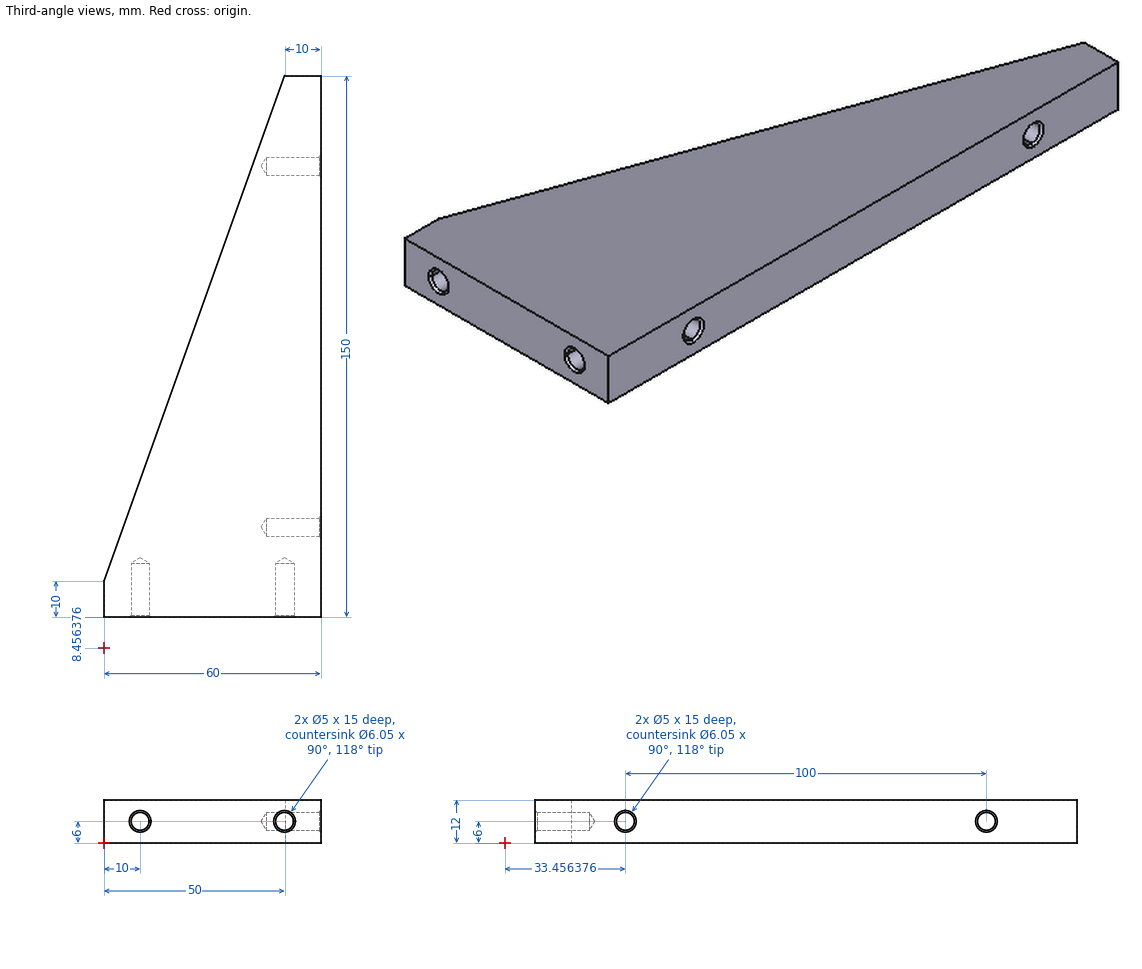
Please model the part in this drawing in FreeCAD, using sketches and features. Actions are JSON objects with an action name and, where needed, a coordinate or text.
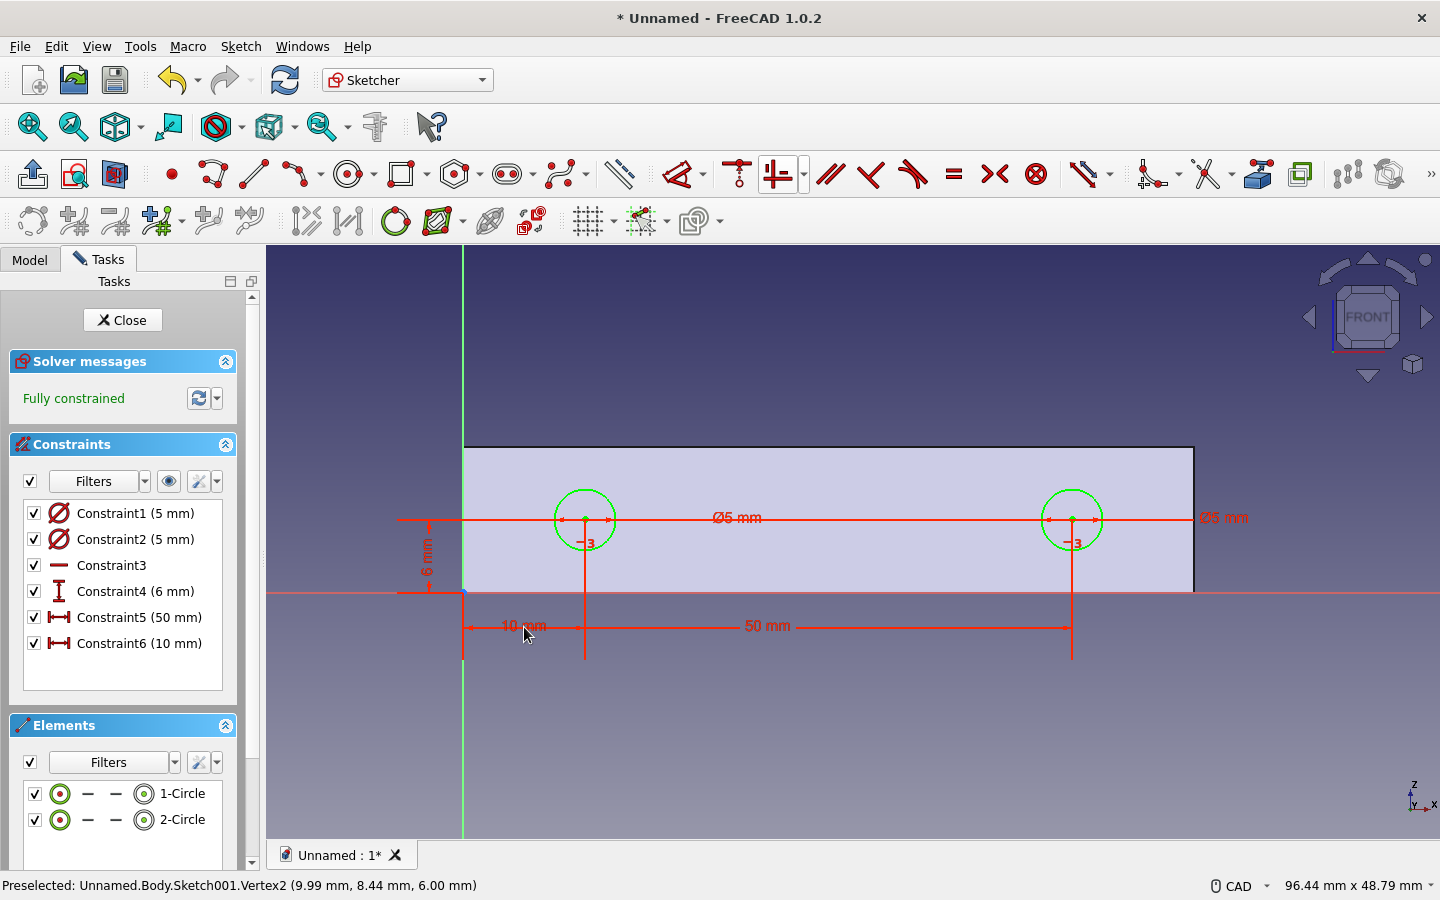
{"action": "left_click", "coordinate": [123, 320]}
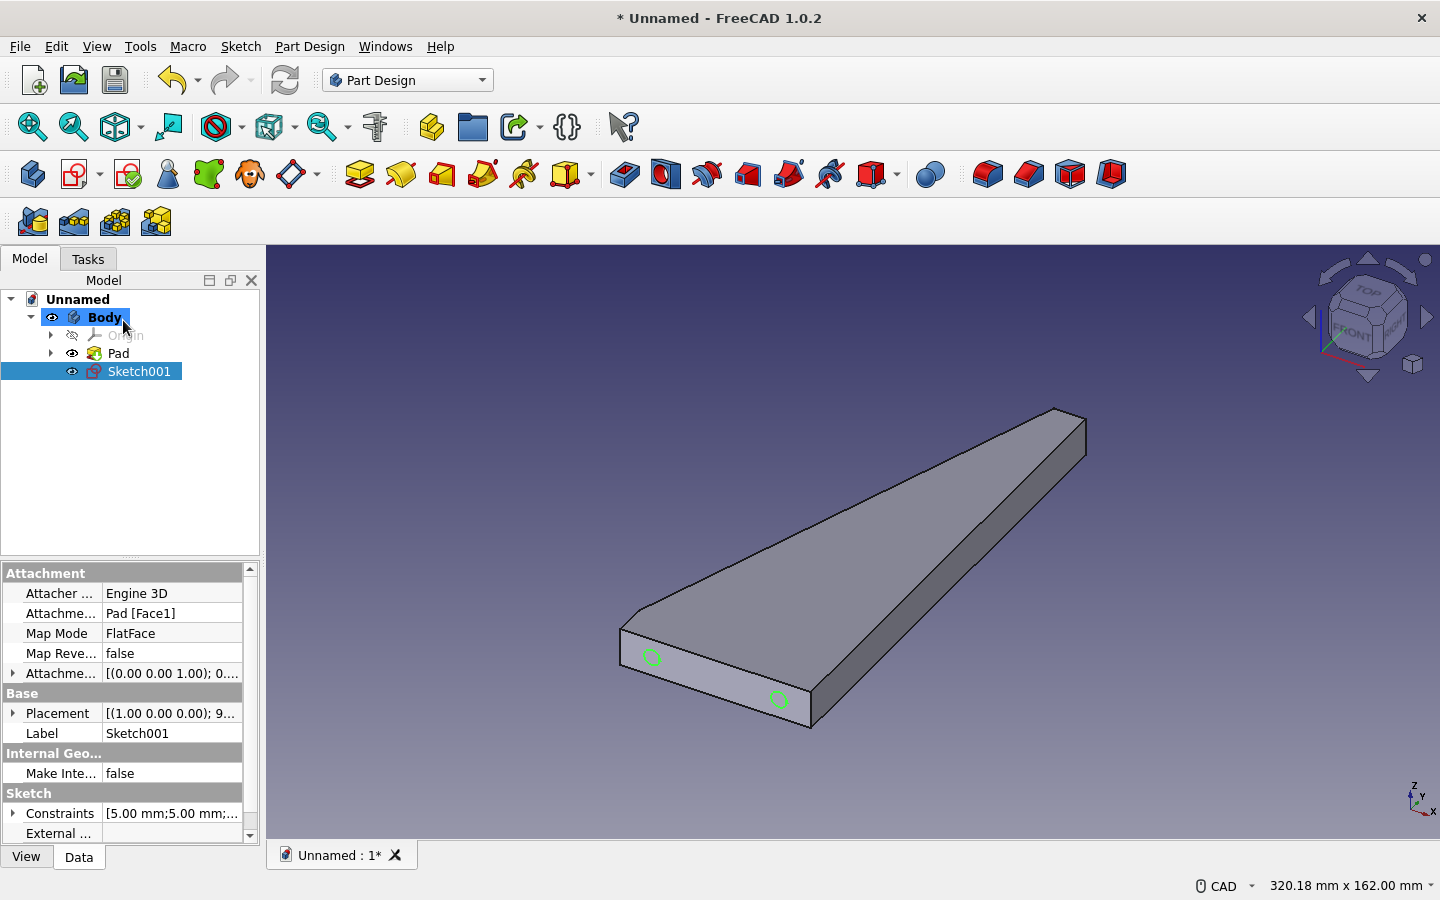
{"action": "left_click", "coordinate": [666, 174]}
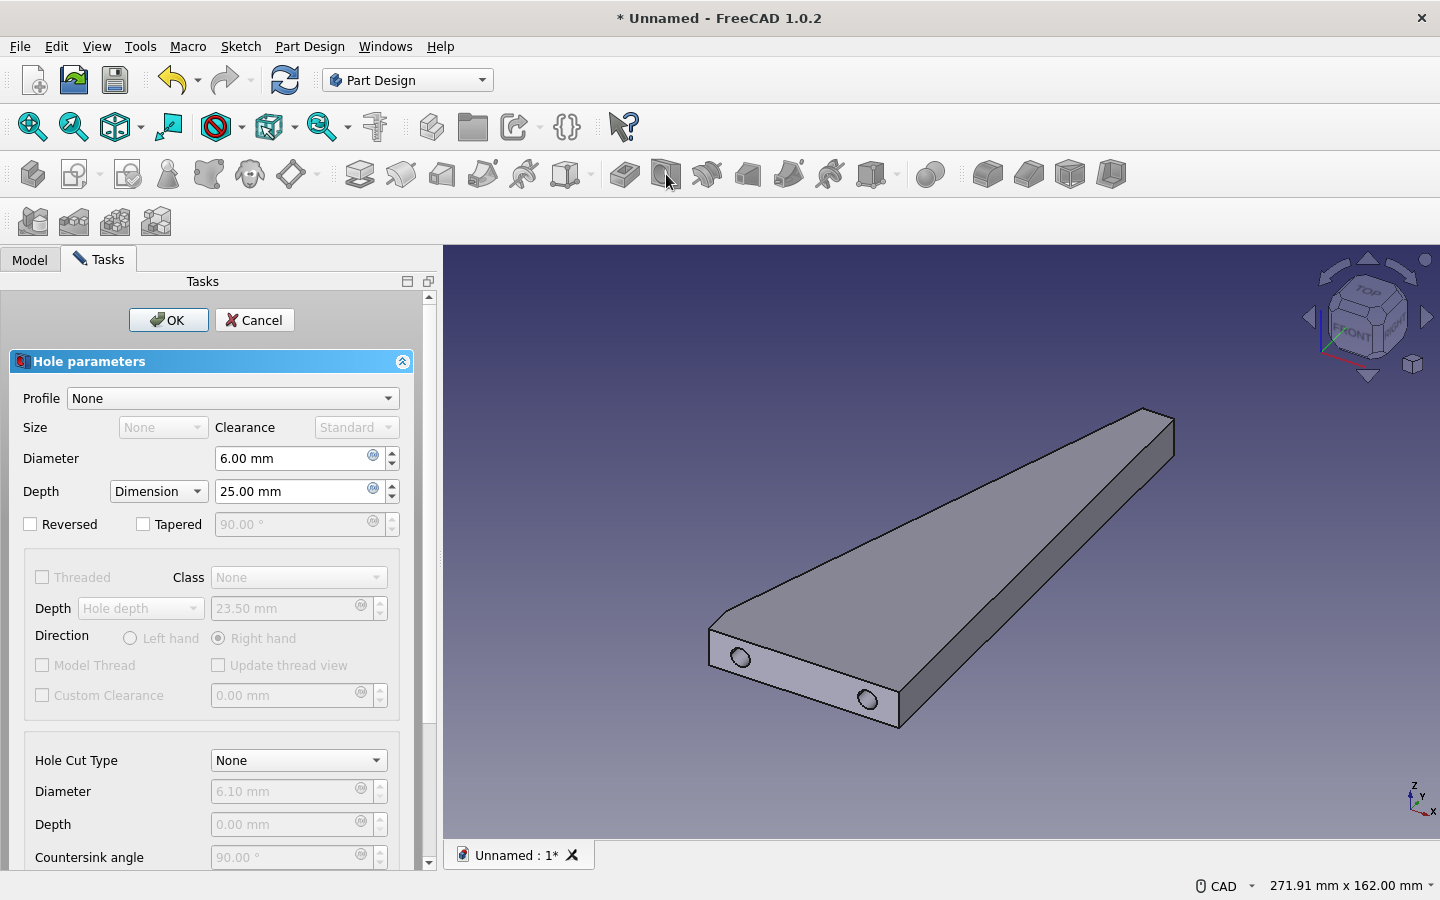
{"action": "triple_click", "coordinate": [300, 458]}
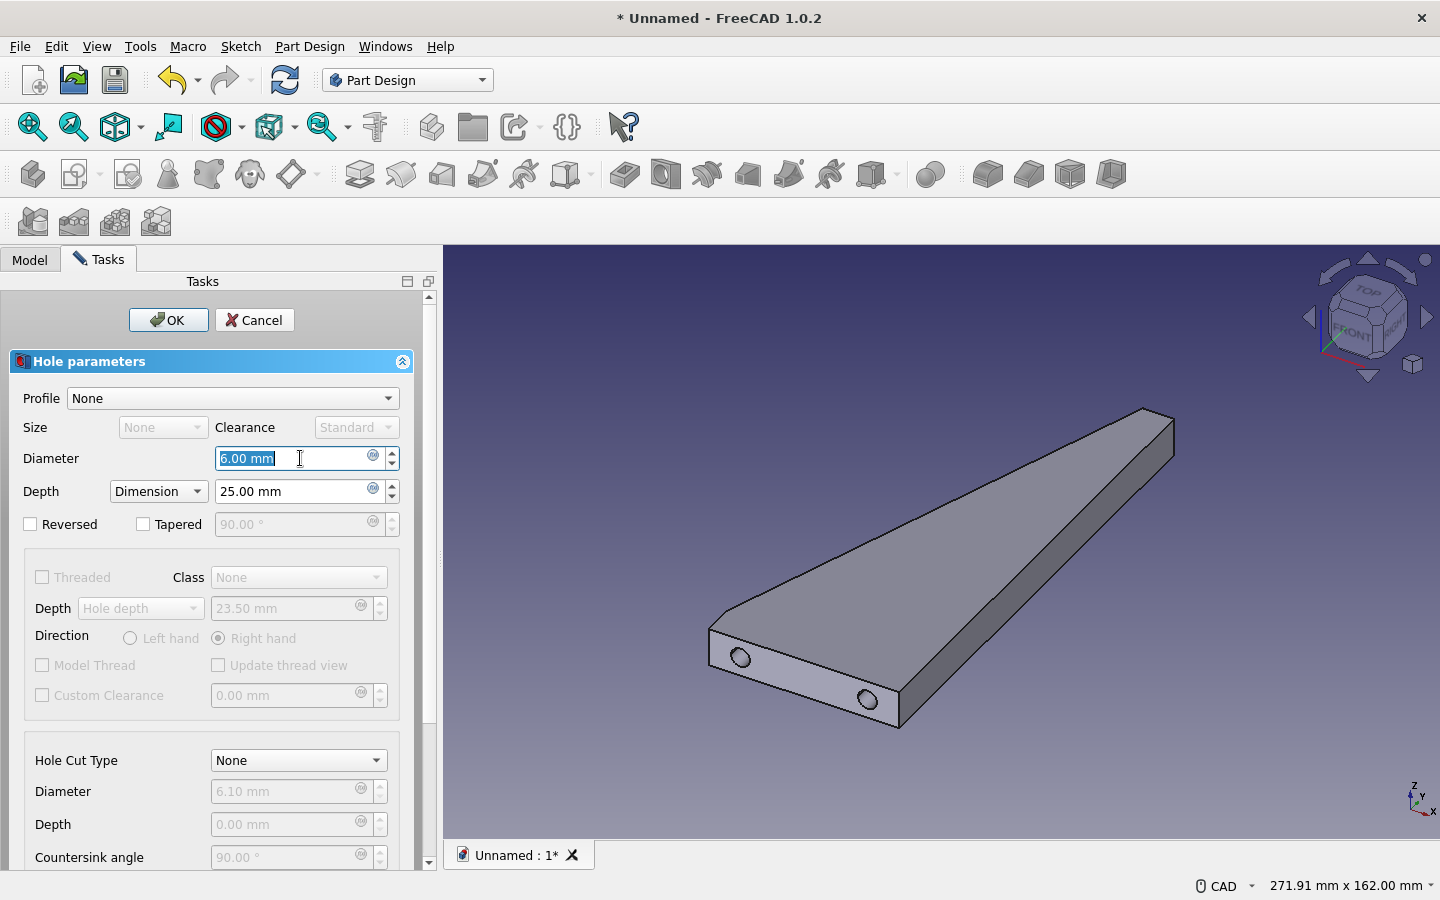
{"action": "type", "text": "5"}
{"action": "key", "text": "Tab"}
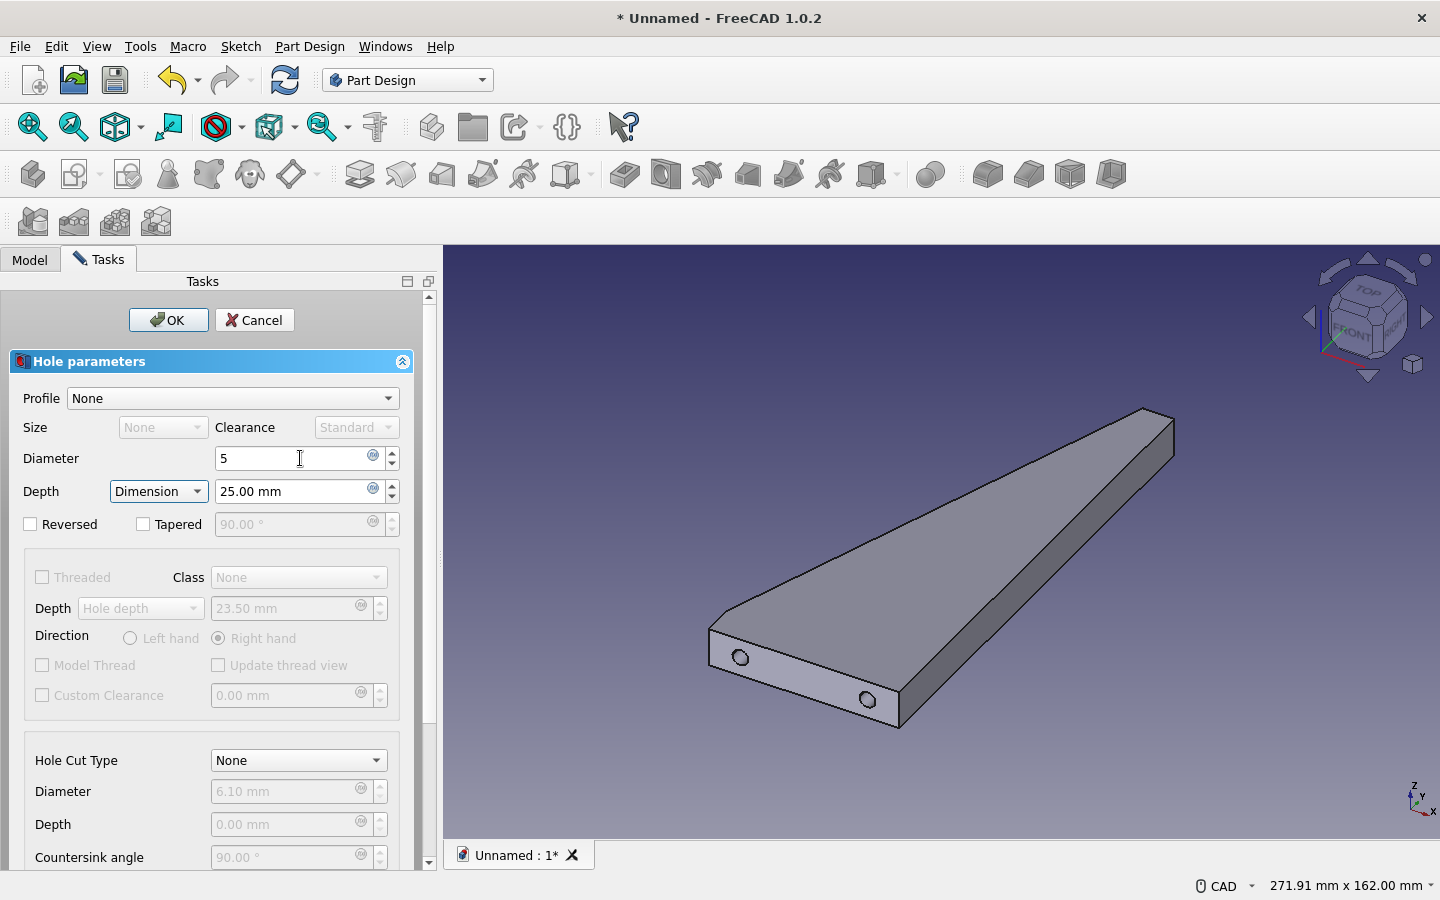
{"action": "triple_click", "coordinate": [300, 492]}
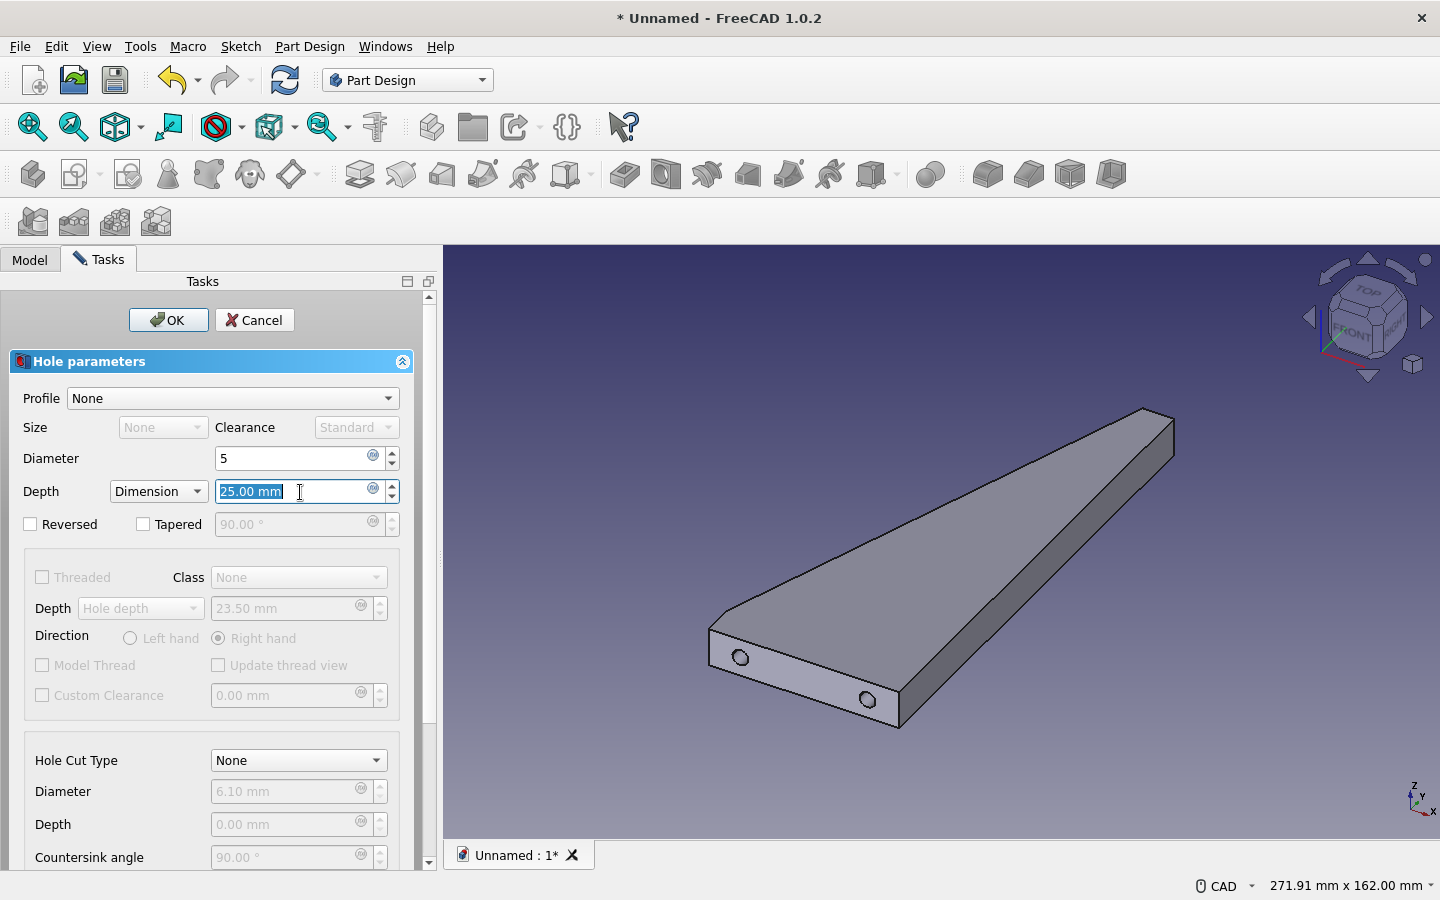
{"action": "type", "text": "15"}
{"action": "key", "text": "Tab"}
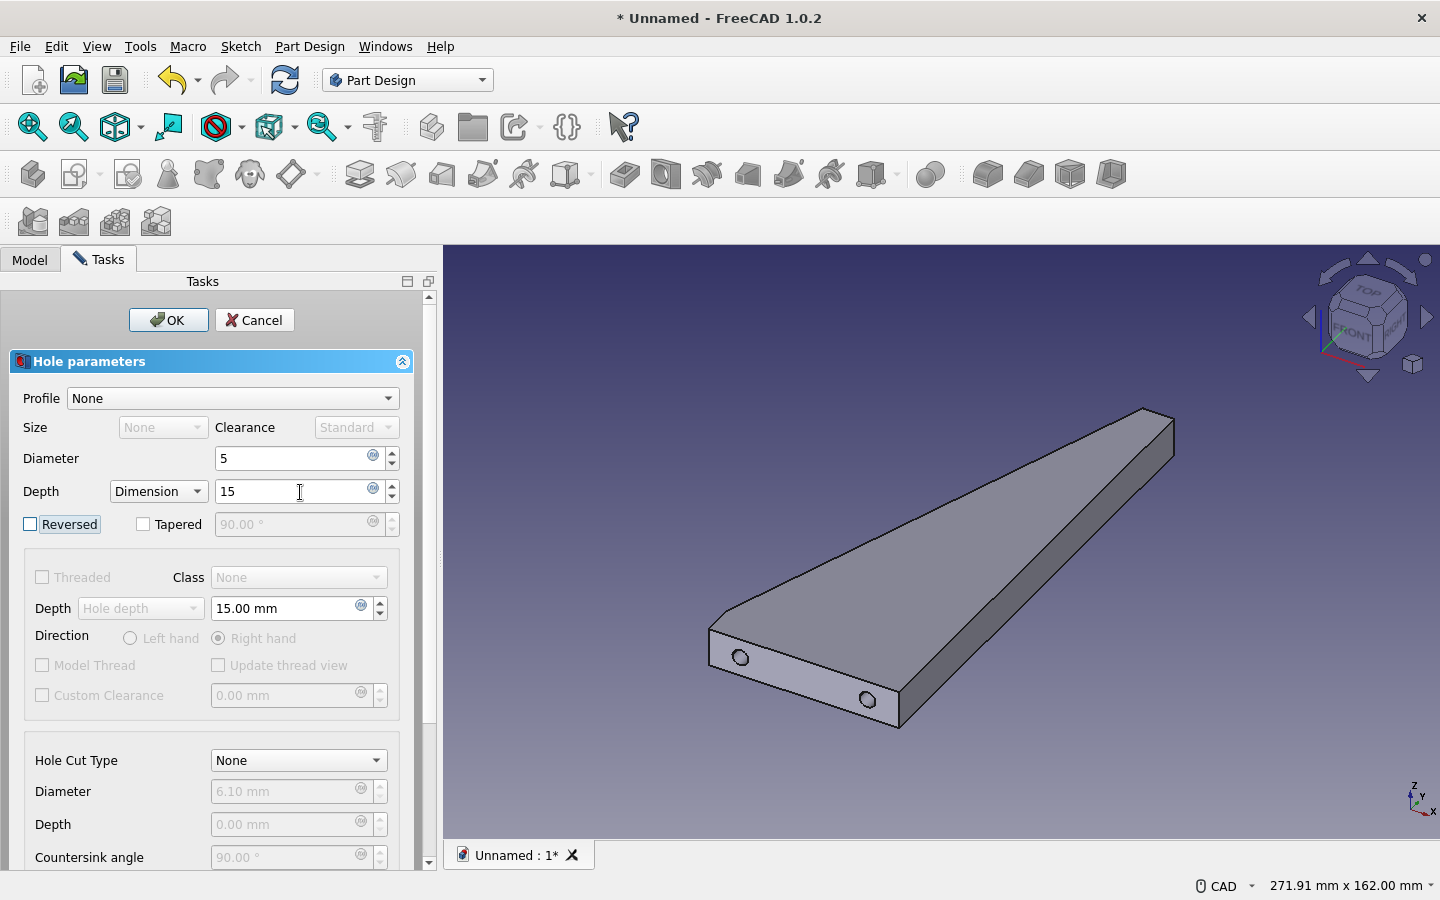
{"action": "left_click", "coordinate": [300, 760]}